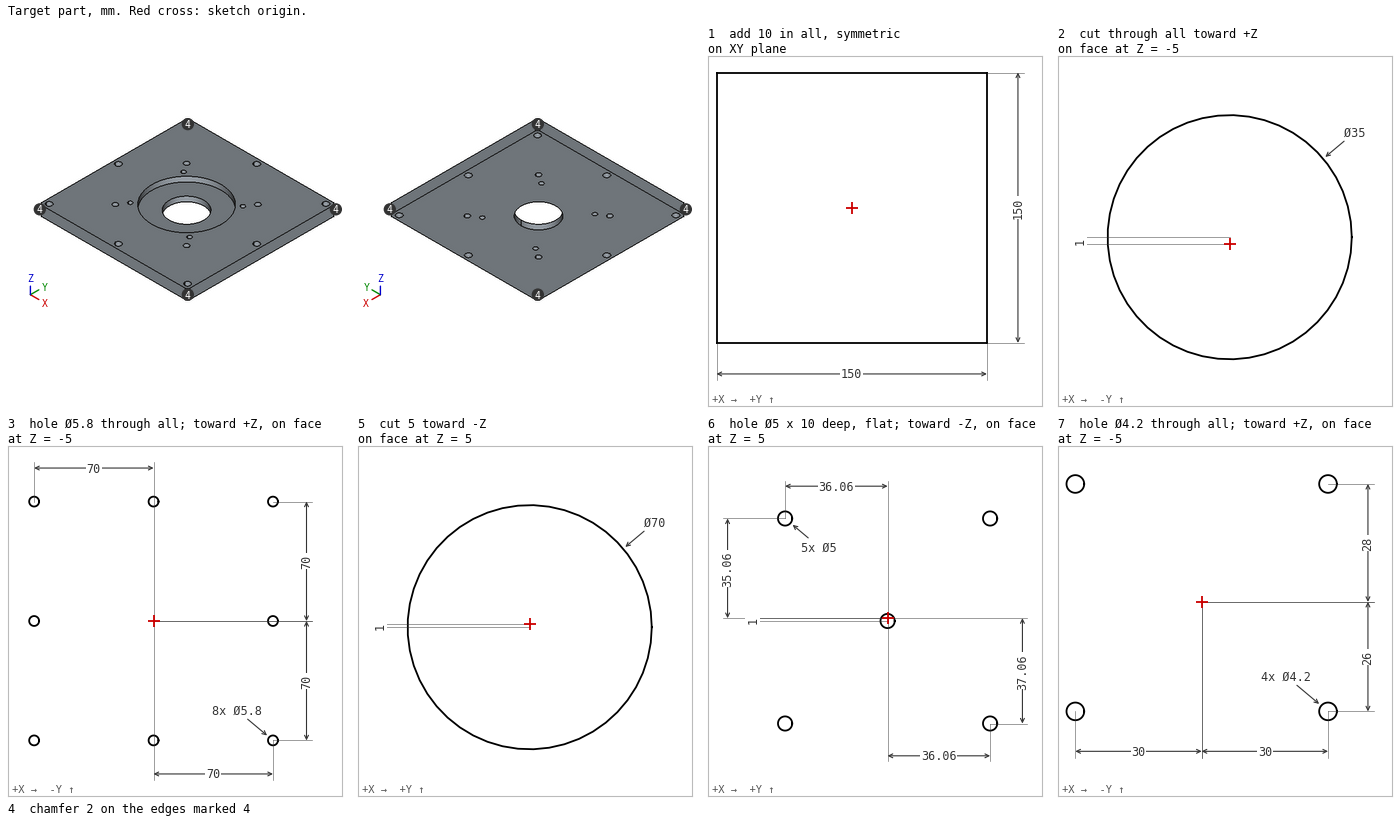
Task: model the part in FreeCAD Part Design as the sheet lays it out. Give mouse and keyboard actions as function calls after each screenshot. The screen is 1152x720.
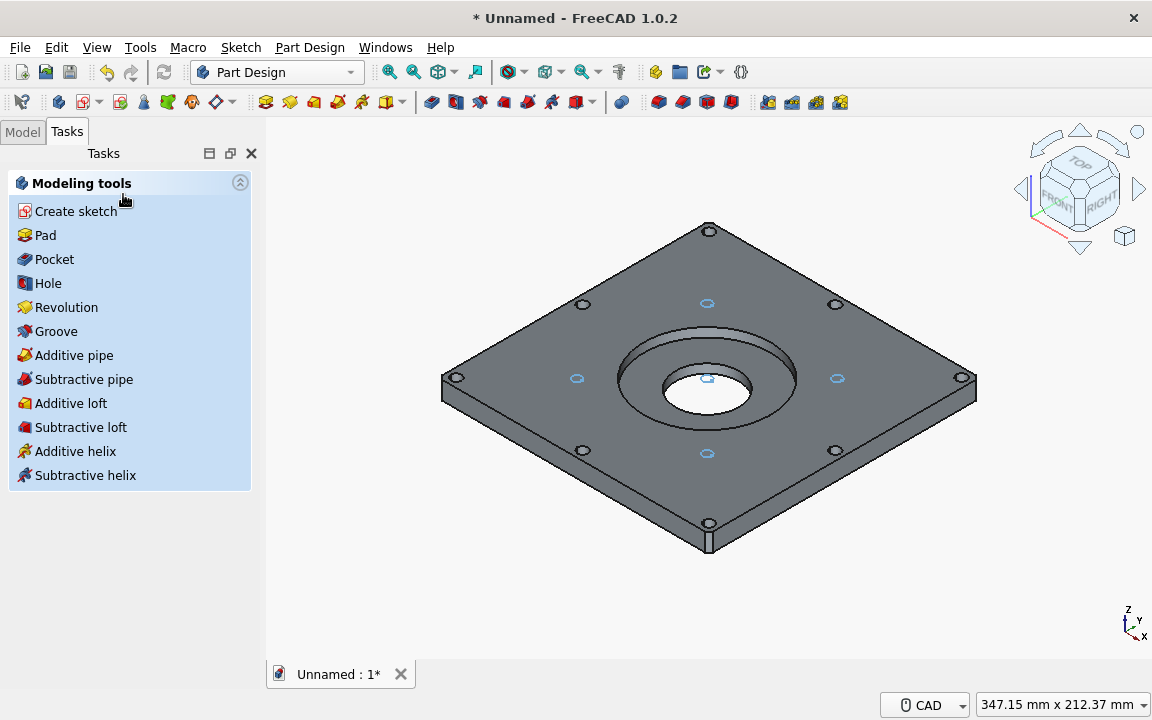
click(456, 102)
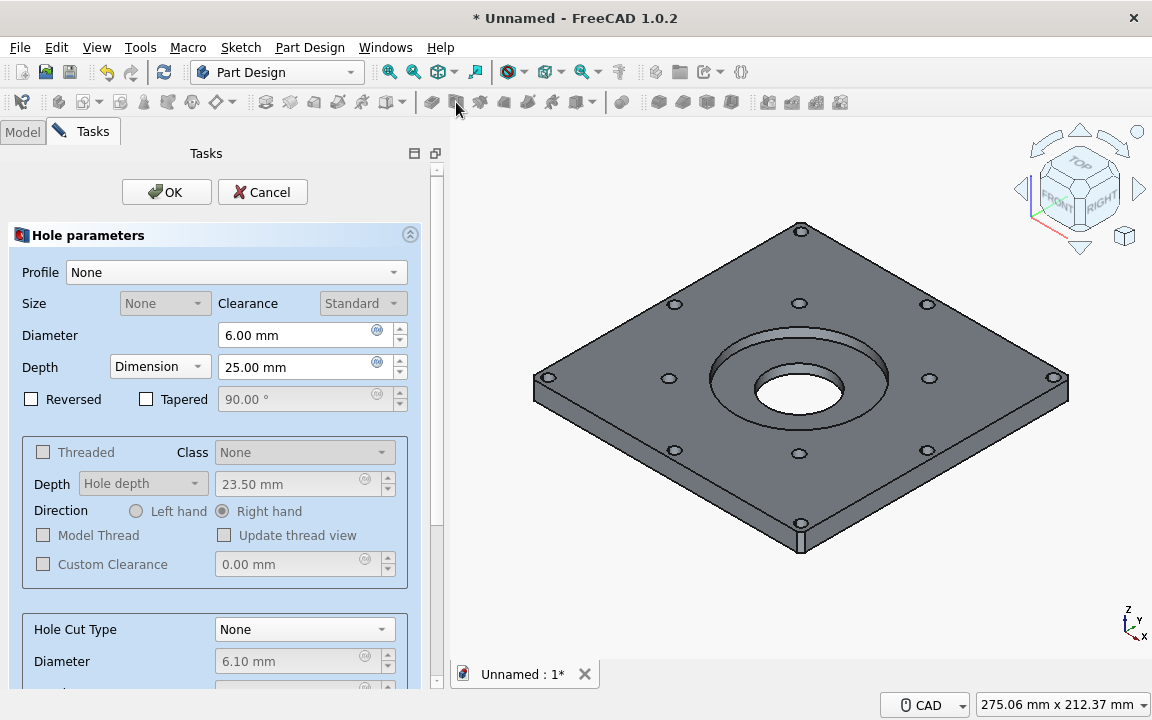
triple_click(305, 335)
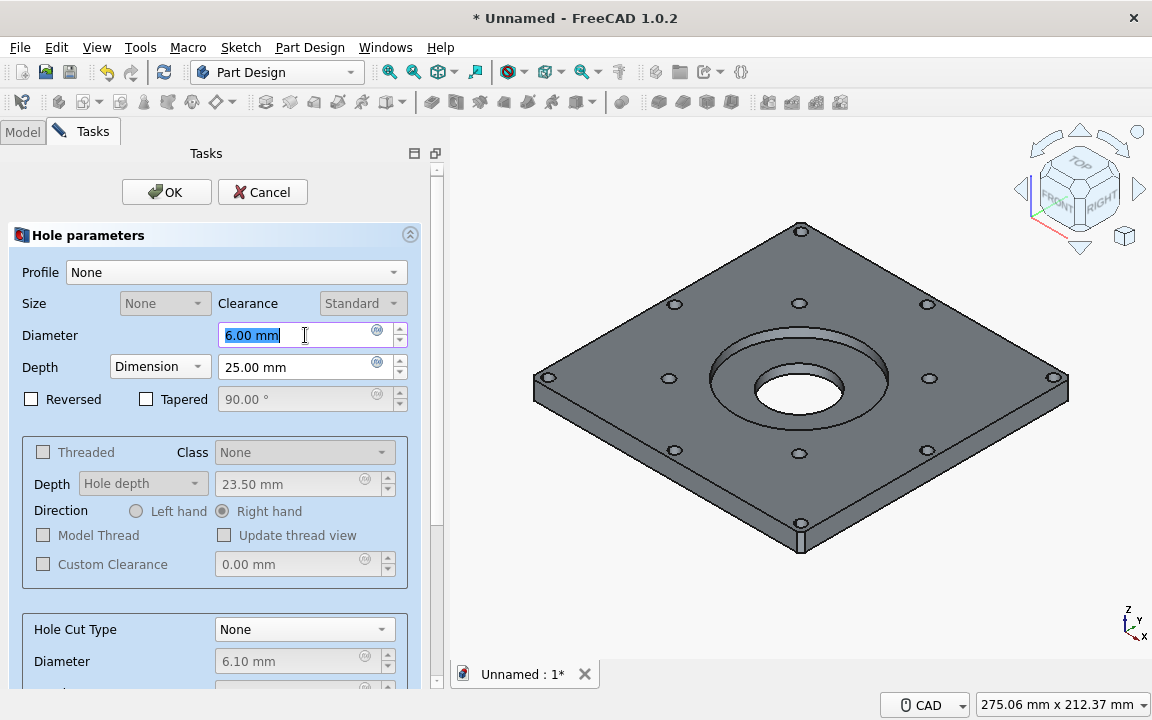
text(5)
key(Tab)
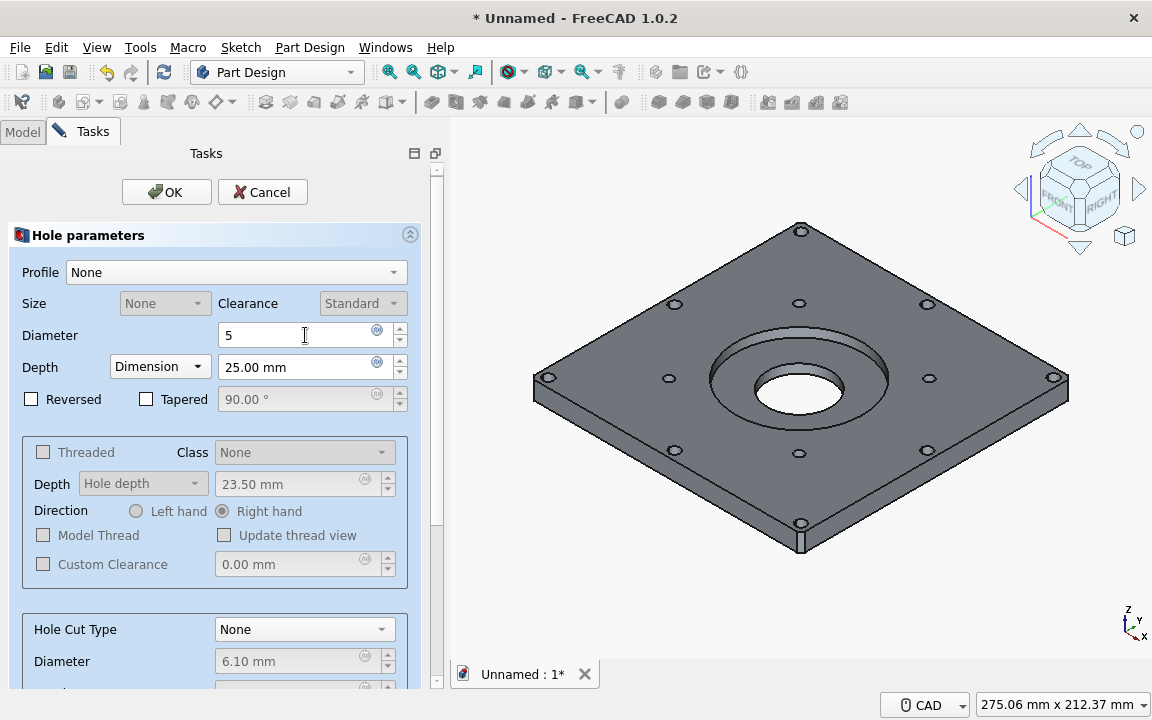
triple_click(305, 367)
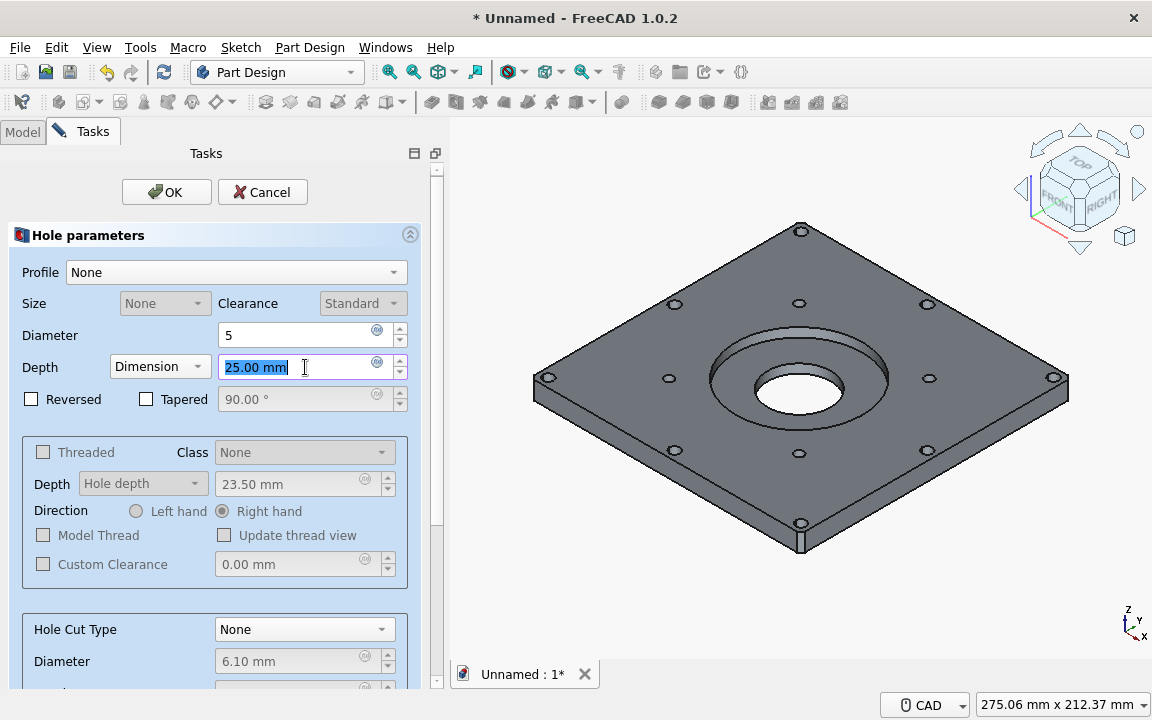
text(10)
key(Tab)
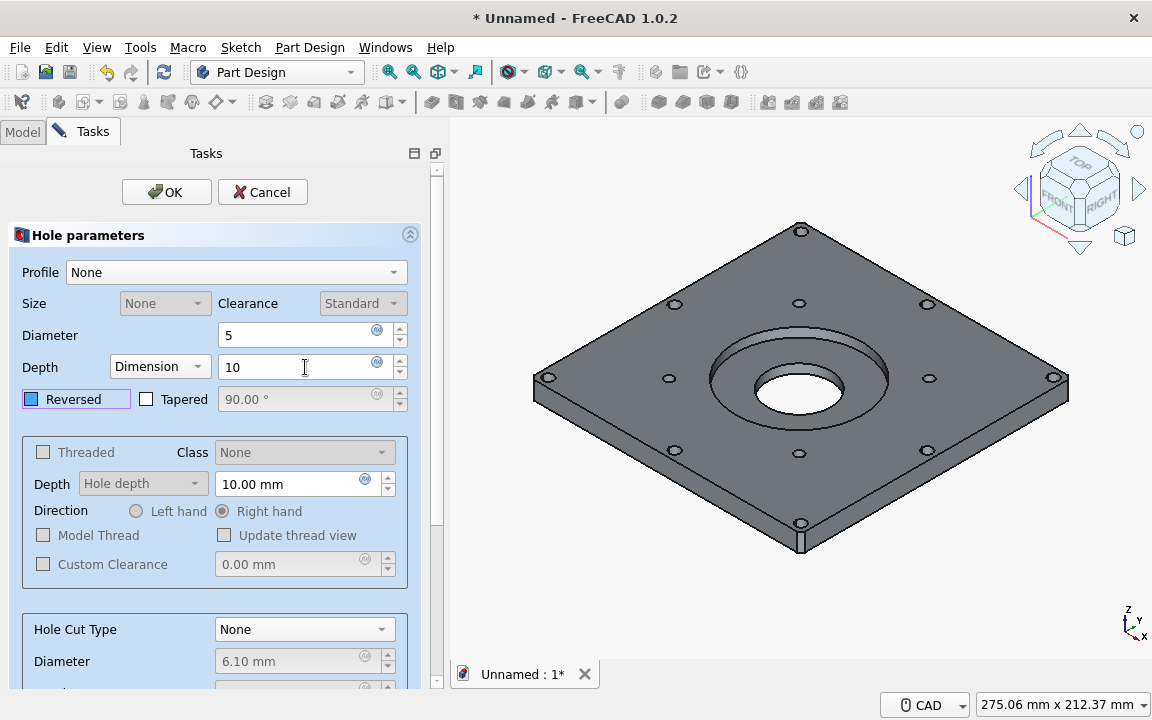
scroll(437, 426, down, 4)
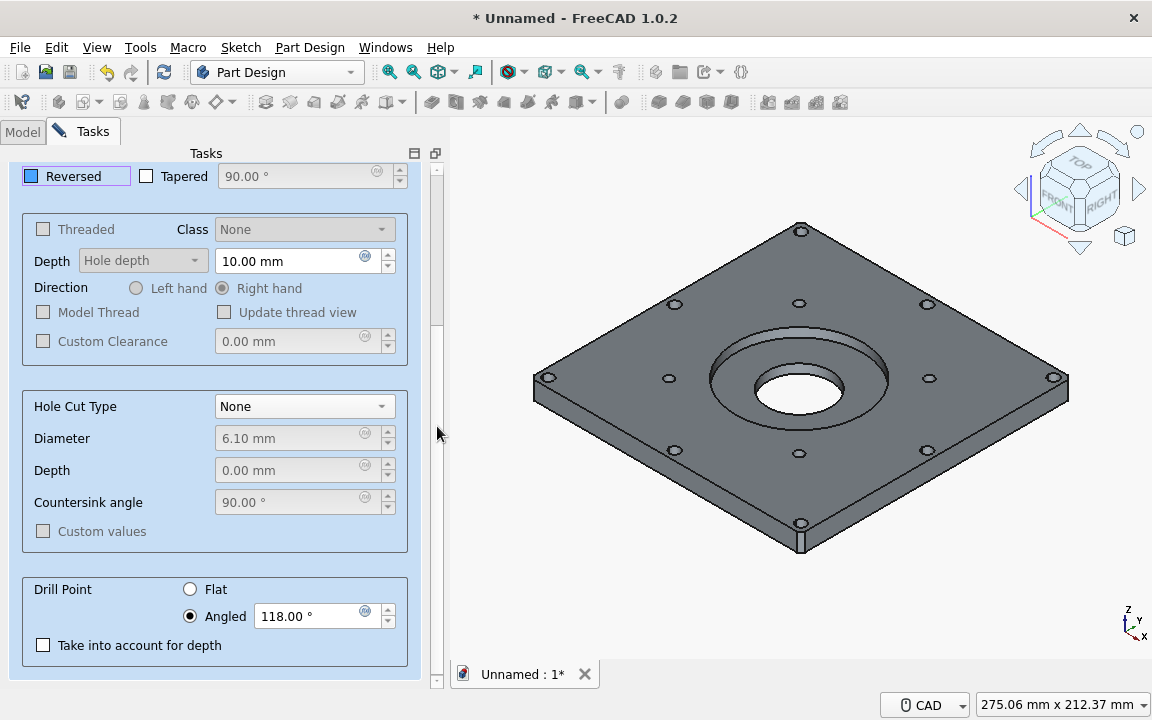
click(191, 589)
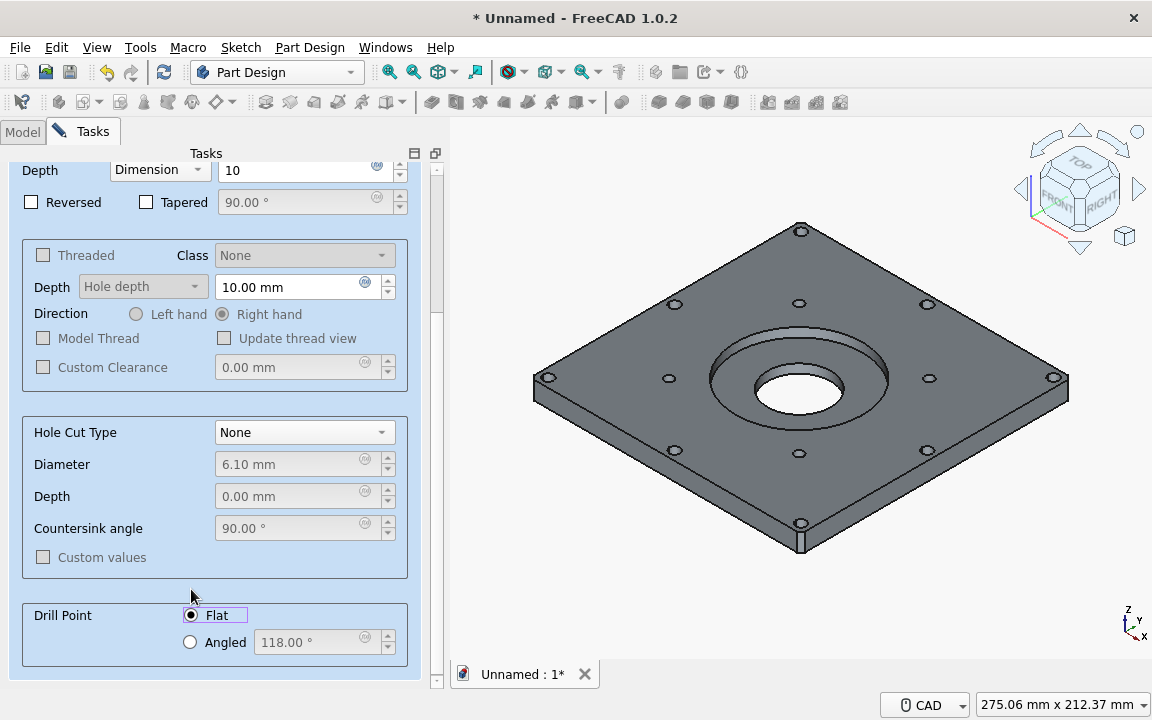
scroll(437, 426, up, 5)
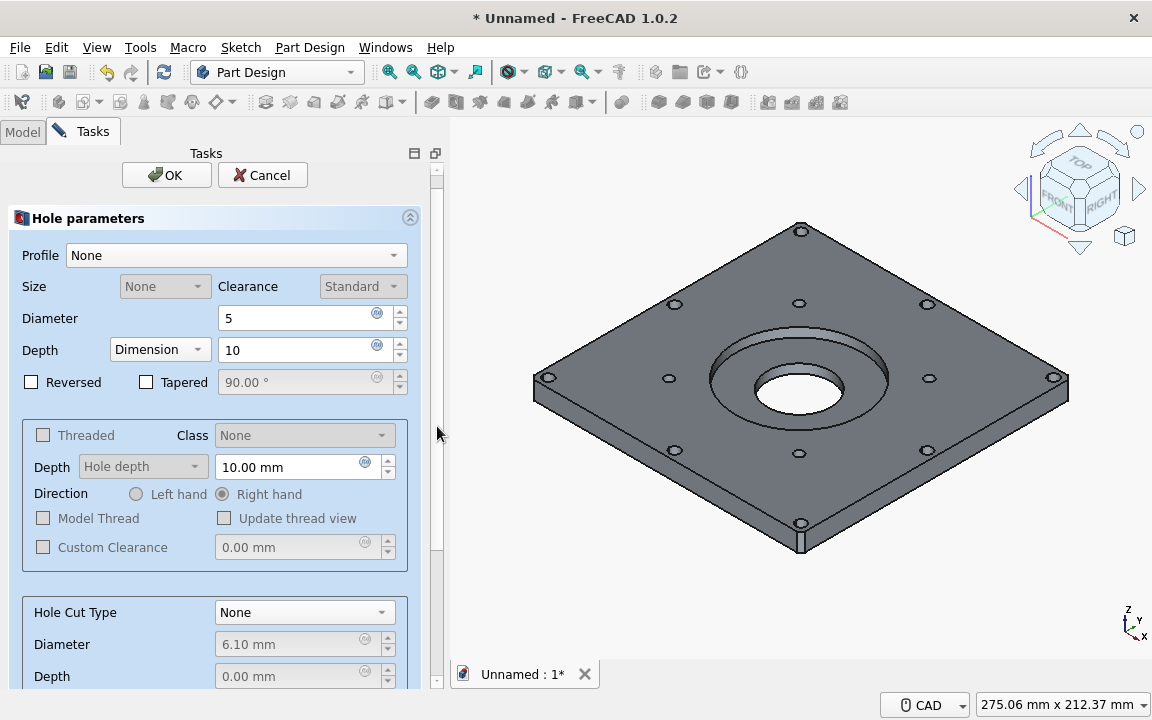
click(167, 192)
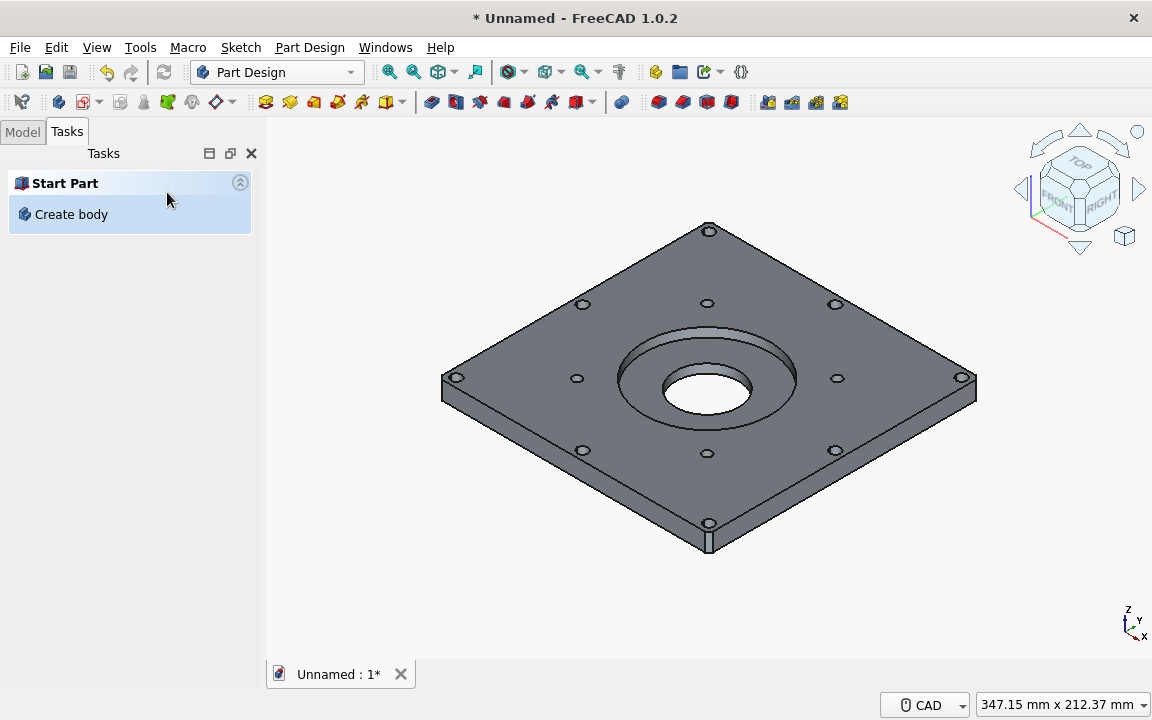
key(5)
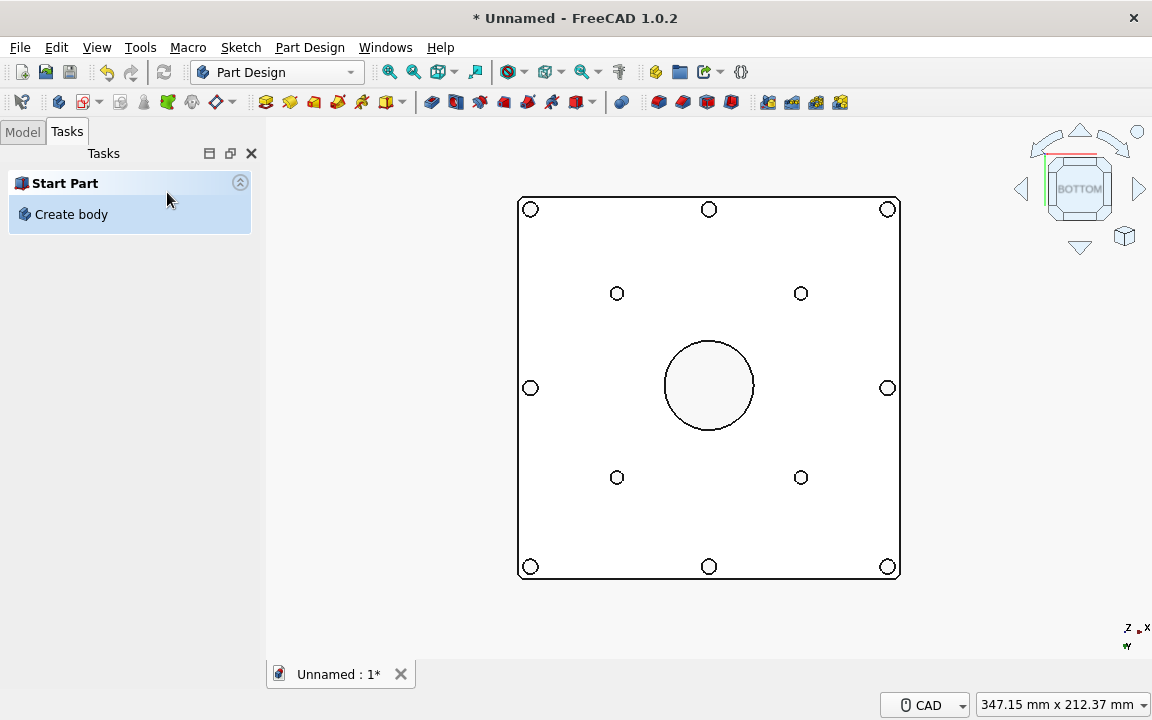
click(709, 278)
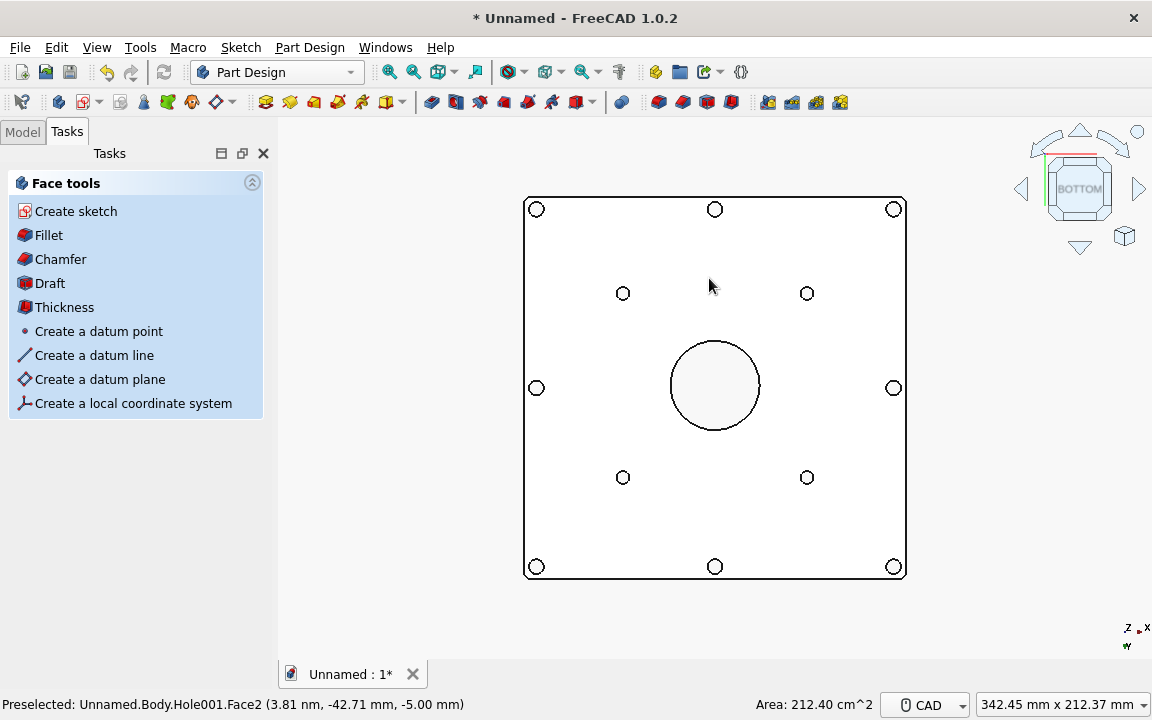
click(84, 102)